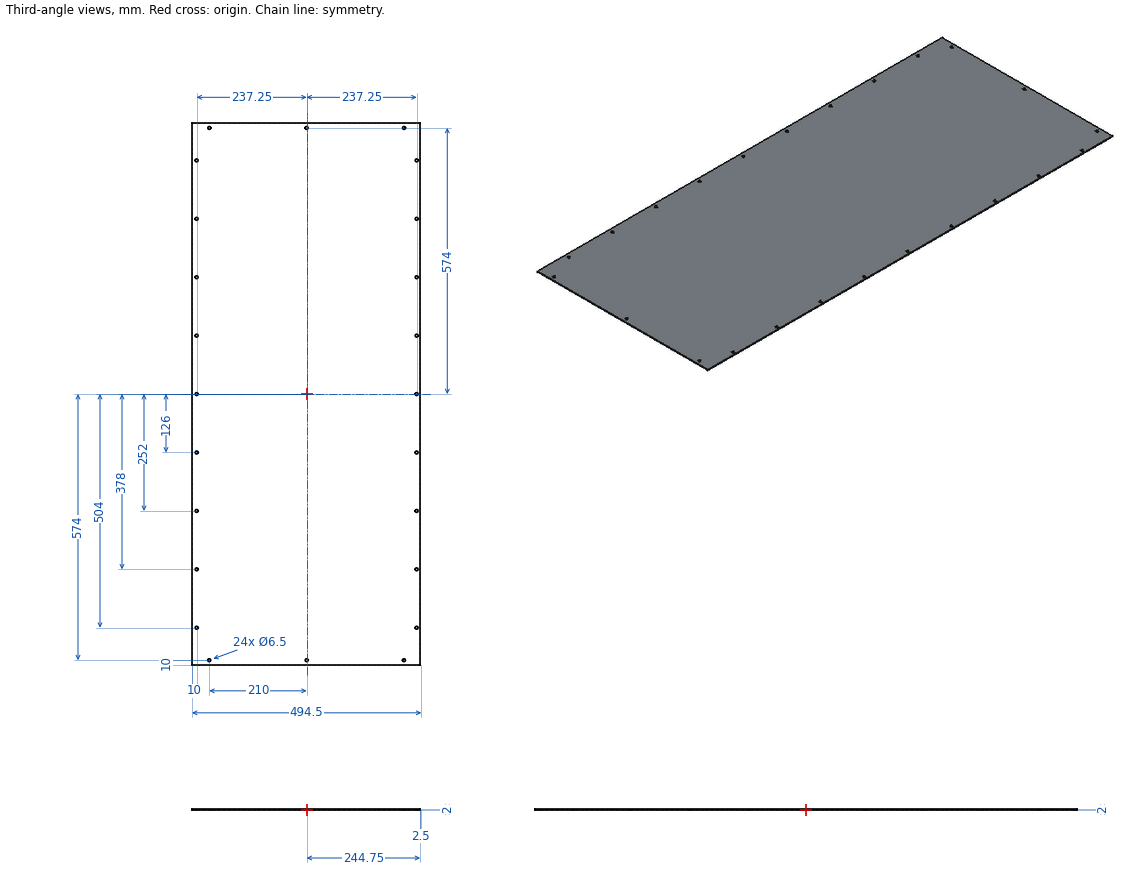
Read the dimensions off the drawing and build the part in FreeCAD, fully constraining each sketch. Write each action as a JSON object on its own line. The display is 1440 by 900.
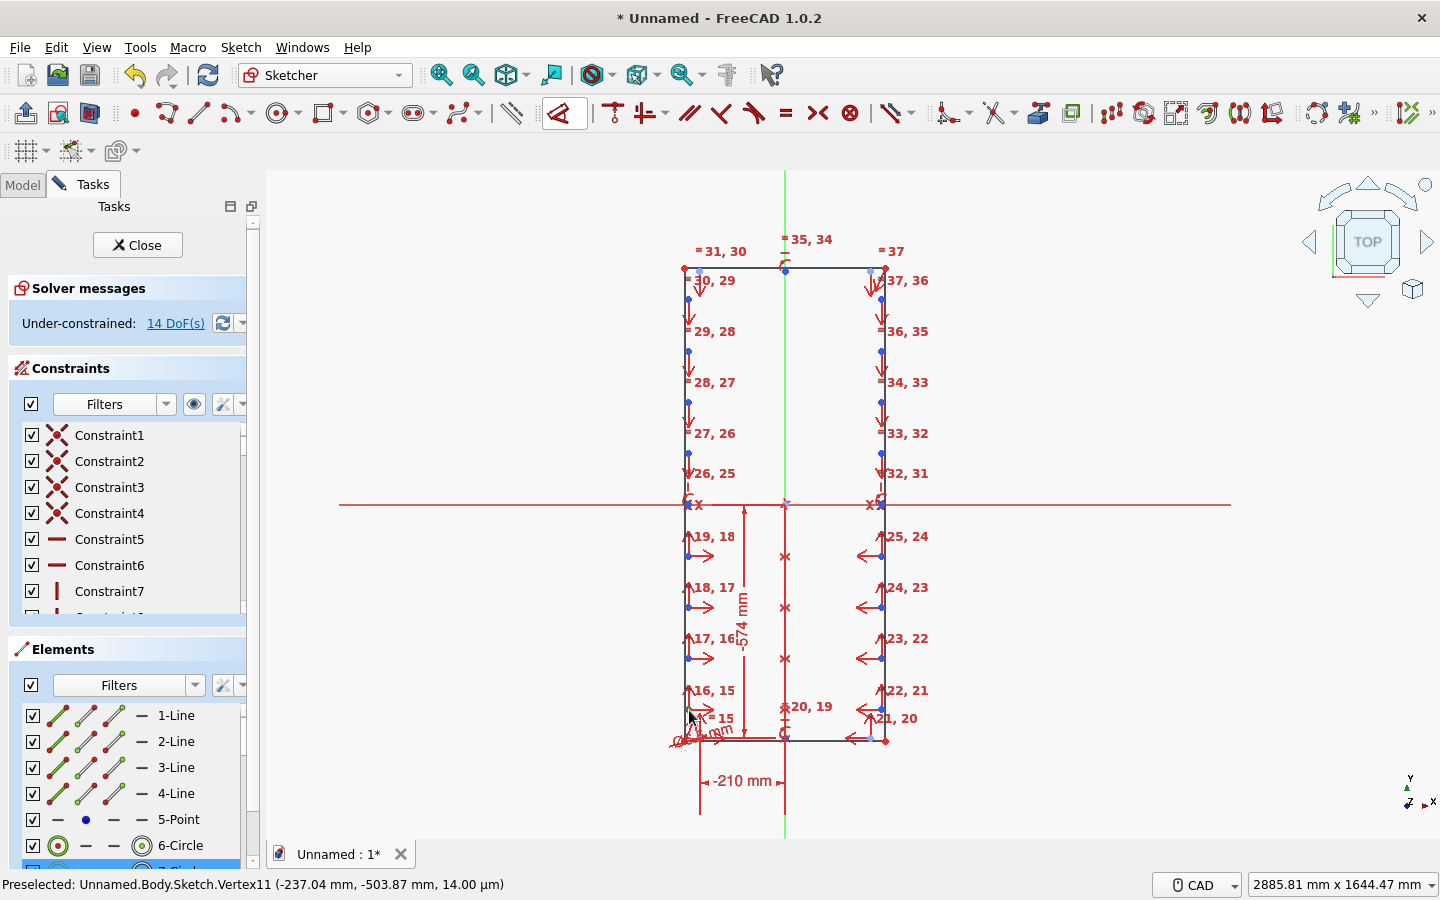
{"action": "key", "text": "i"}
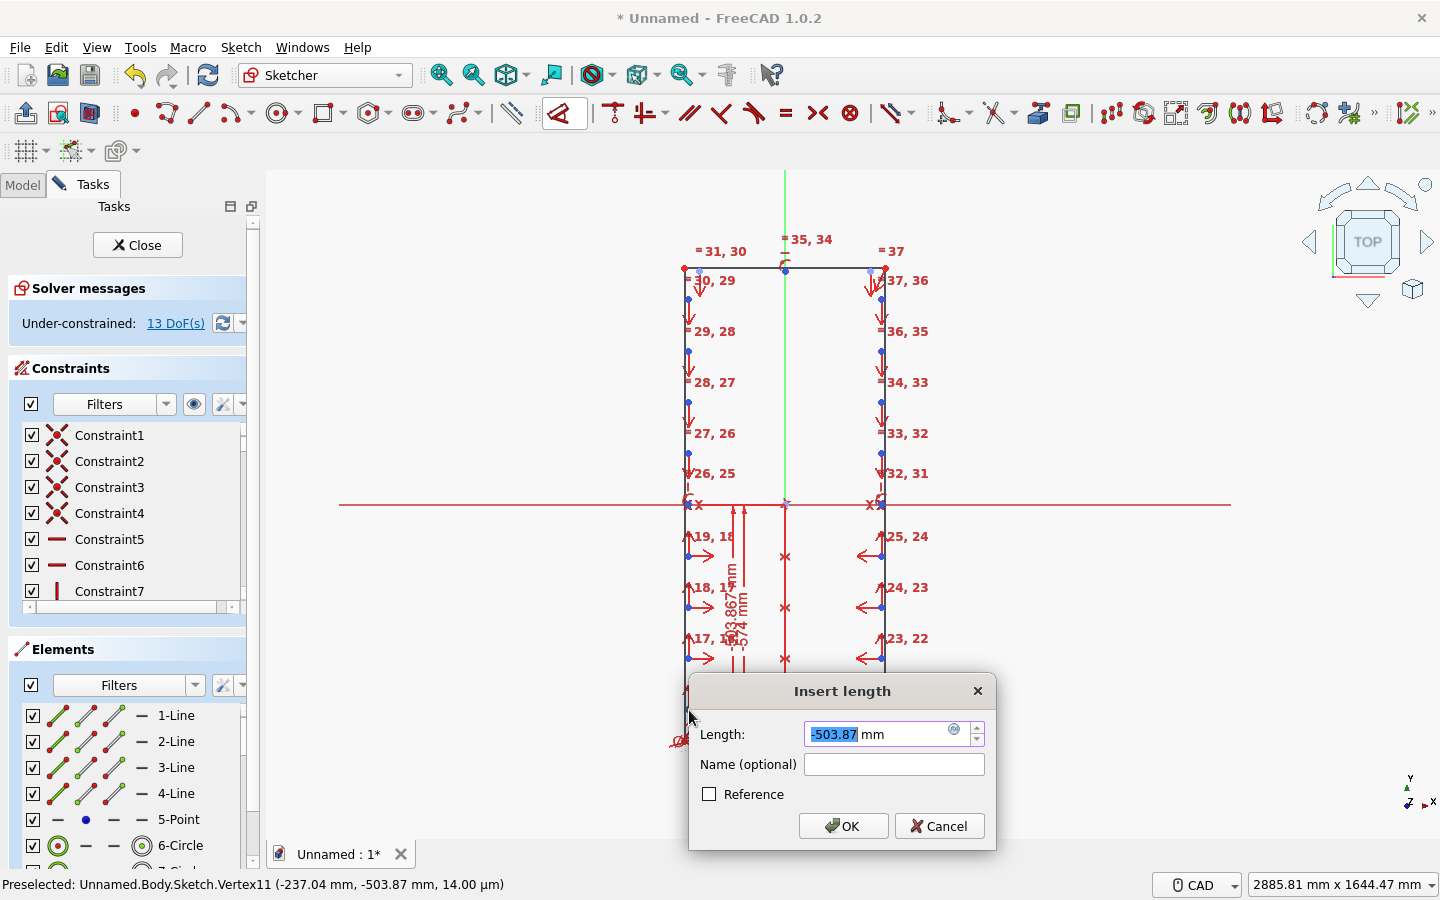
{"action": "type", "text": "-504"}
{"action": "key", "text": "Return"}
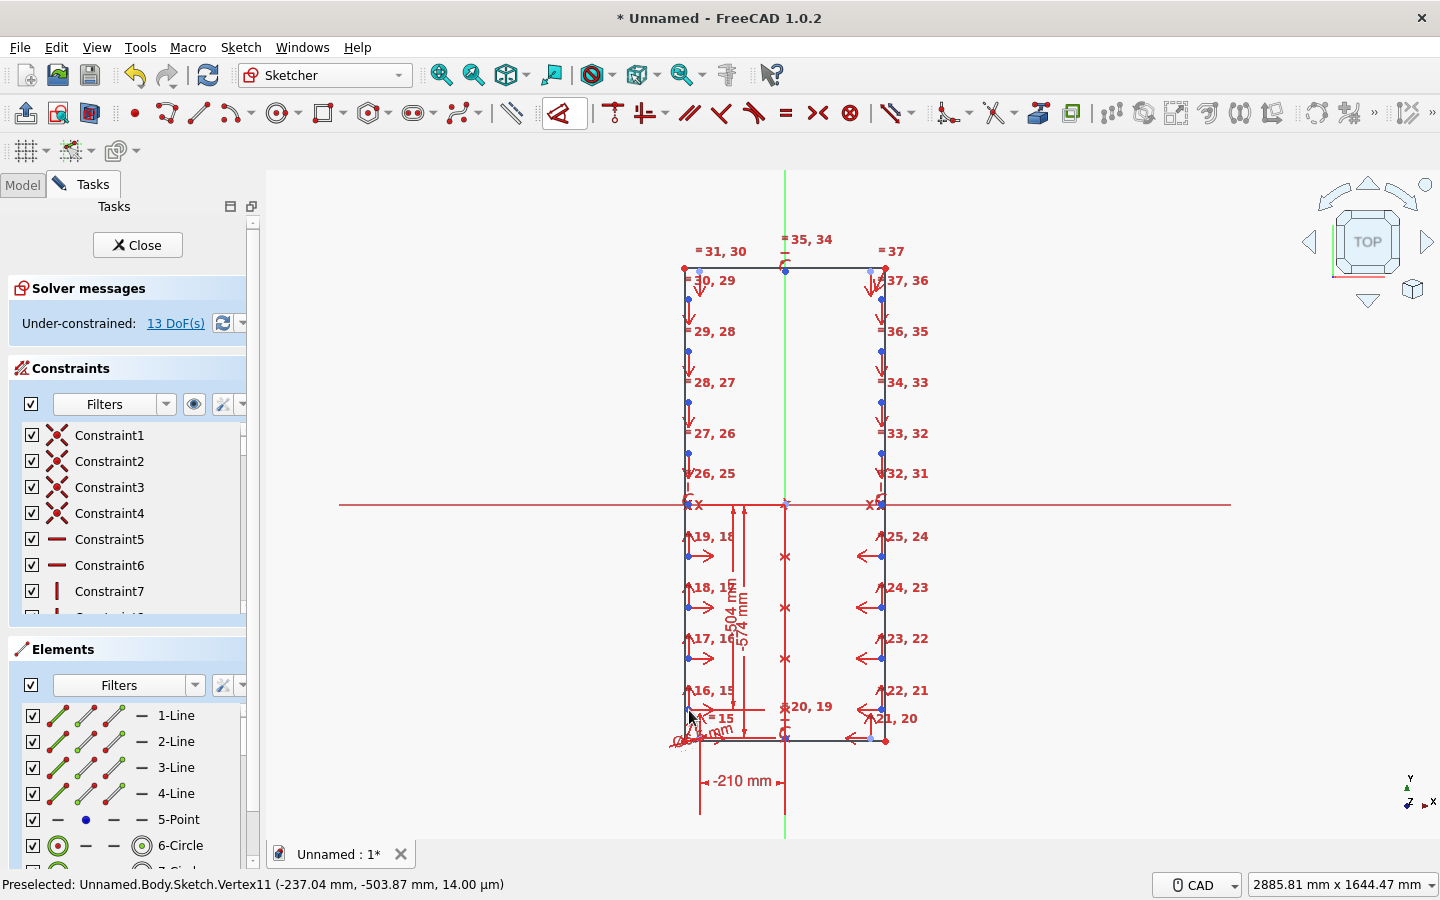
{"action": "left_click", "coordinate": [689, 659]}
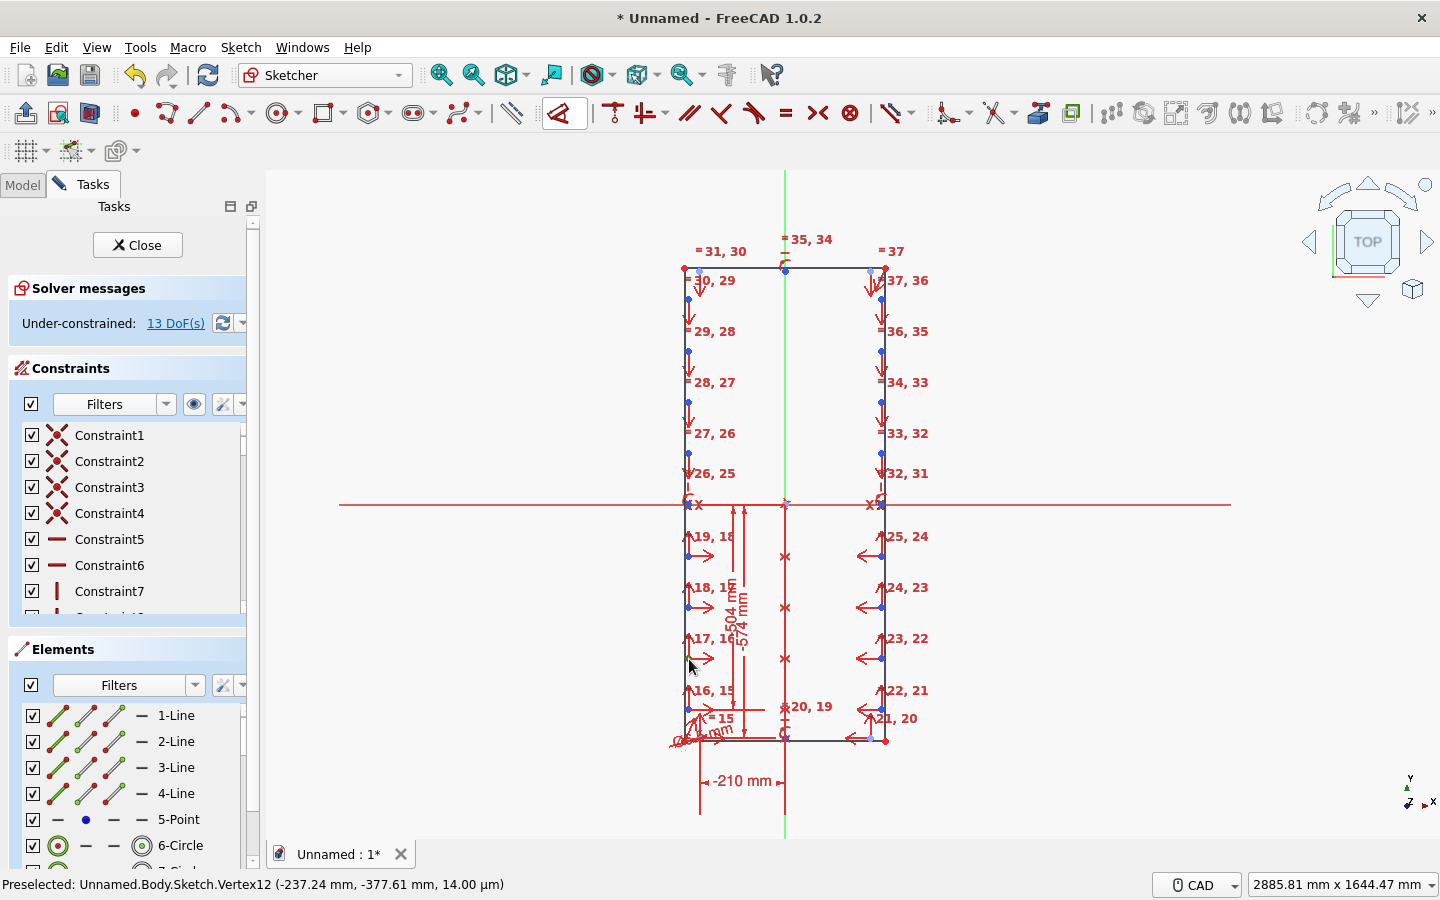
{"action": "key", "text": "i"}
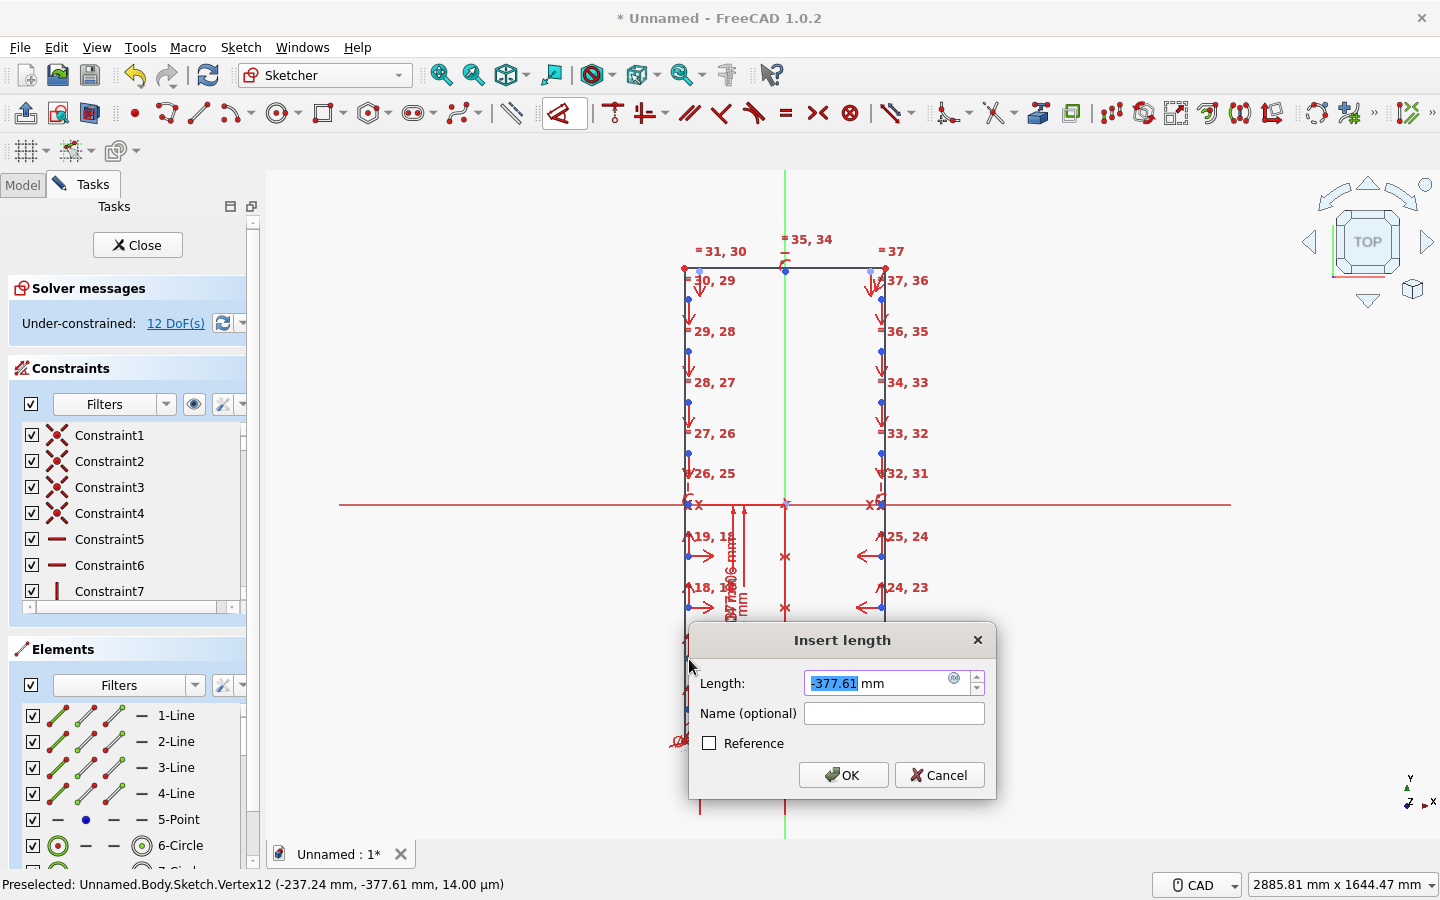
{"action": "type", "text": "-378"}
{"action": "key", "text": "Return"}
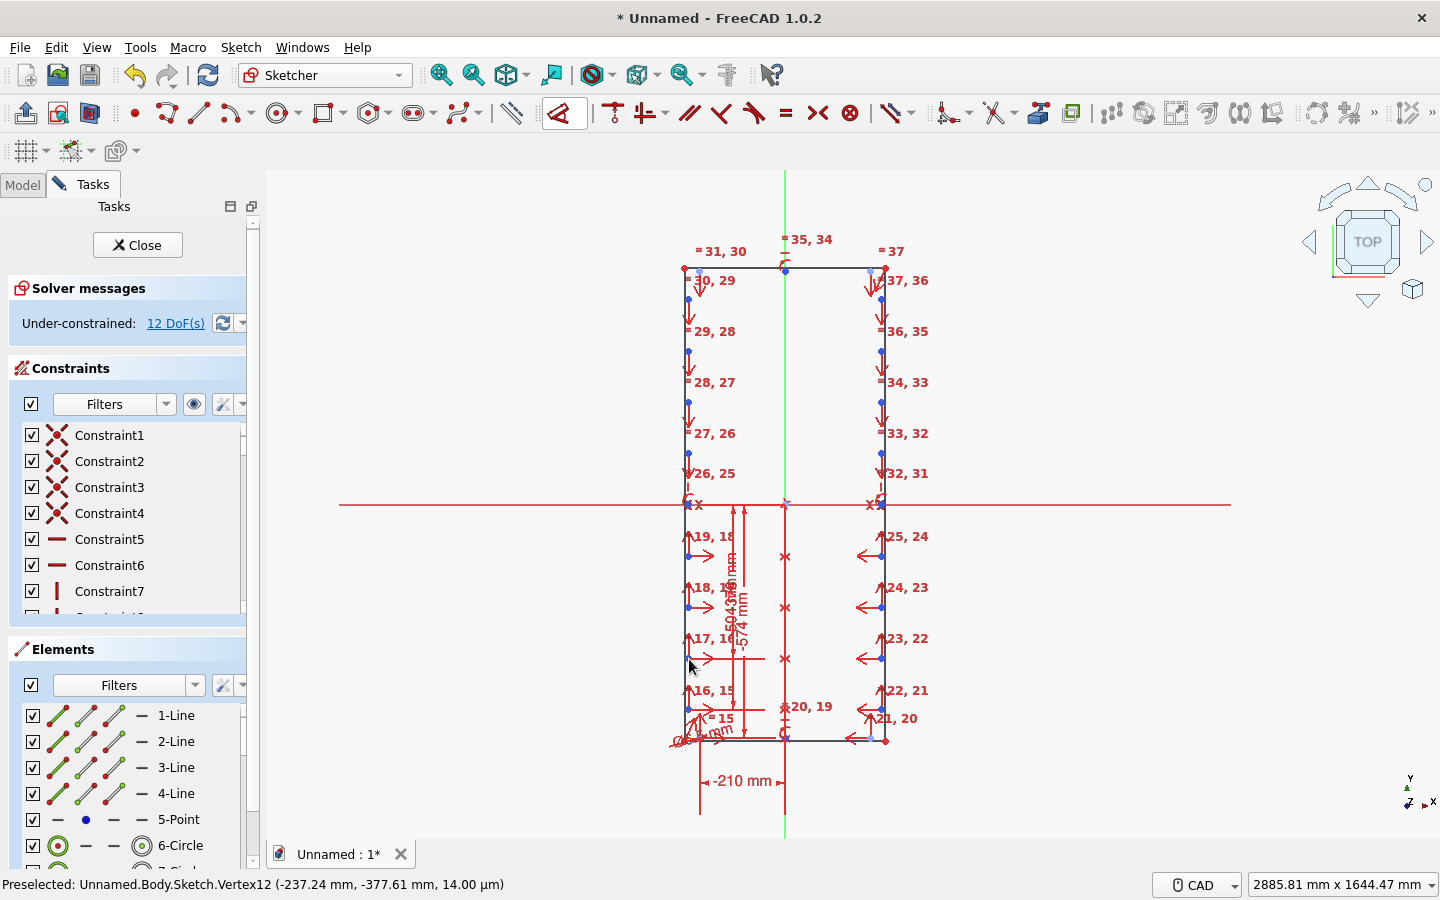
{"action": "left_click", "coordinate": [689, 608]}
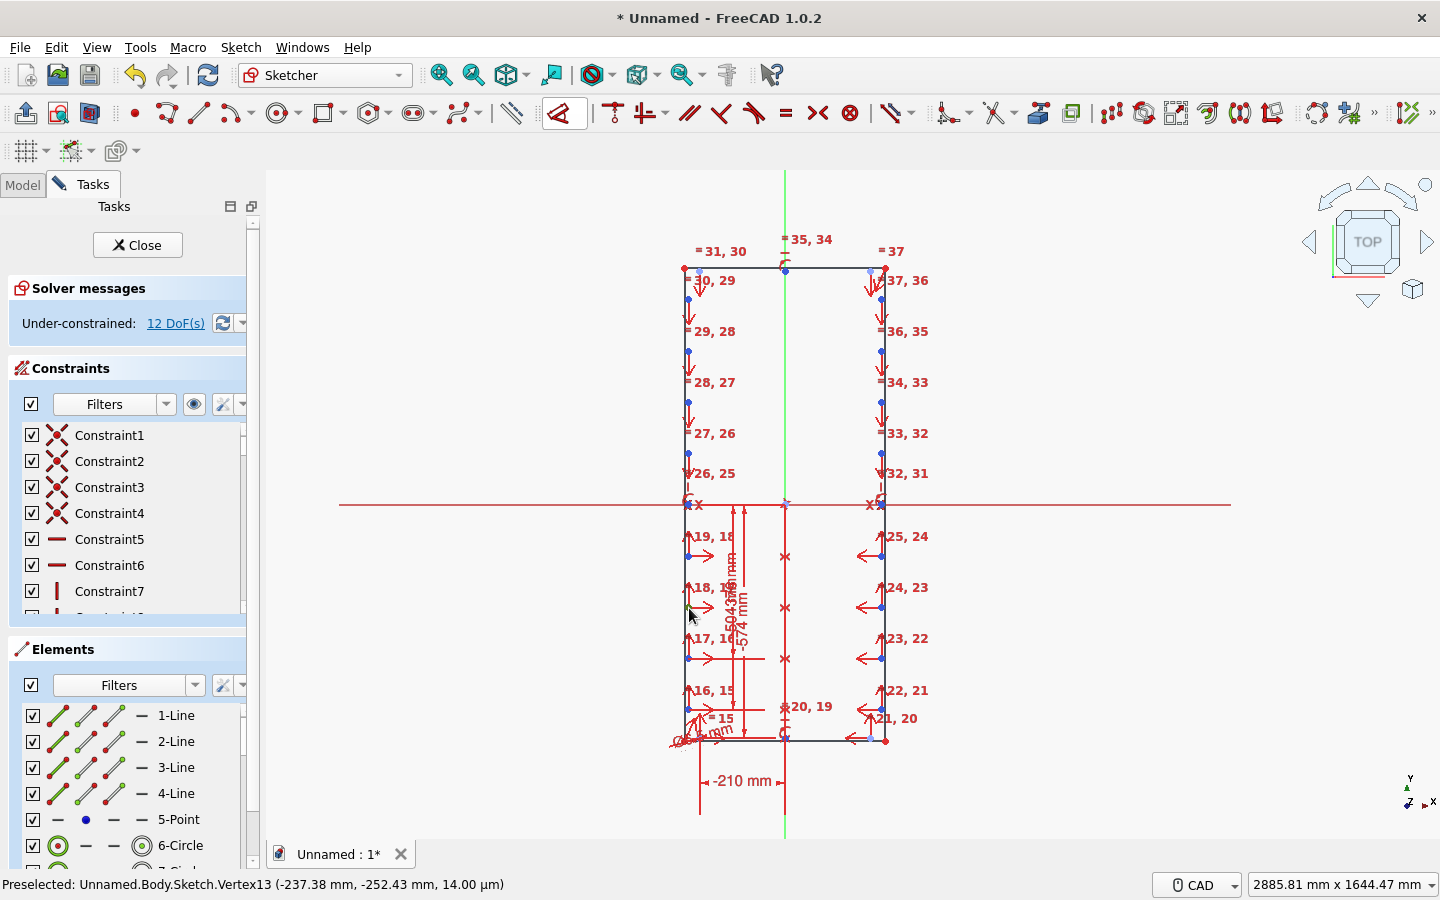
{"action": "key", "text": "i"}